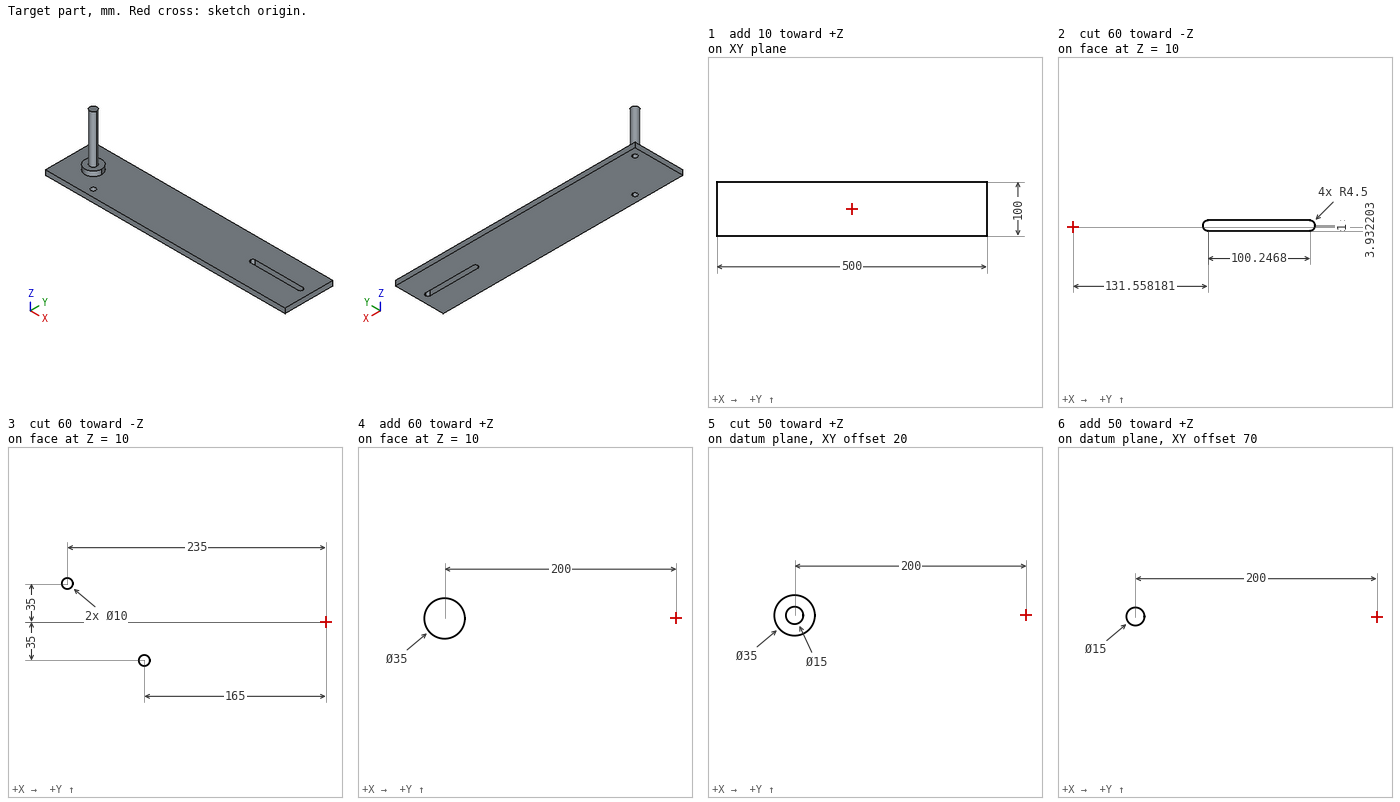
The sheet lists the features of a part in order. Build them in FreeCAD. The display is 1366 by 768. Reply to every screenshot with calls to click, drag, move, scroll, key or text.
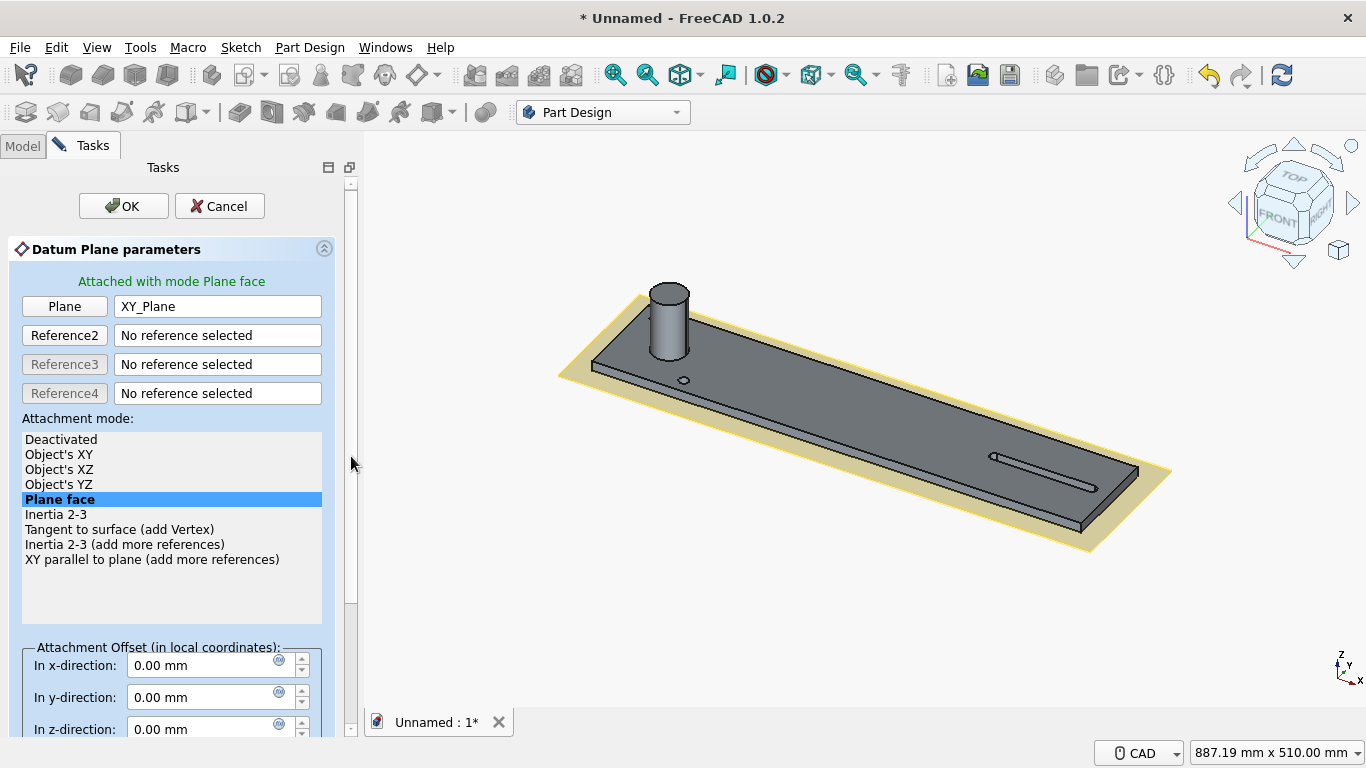
triple_click(210, 609)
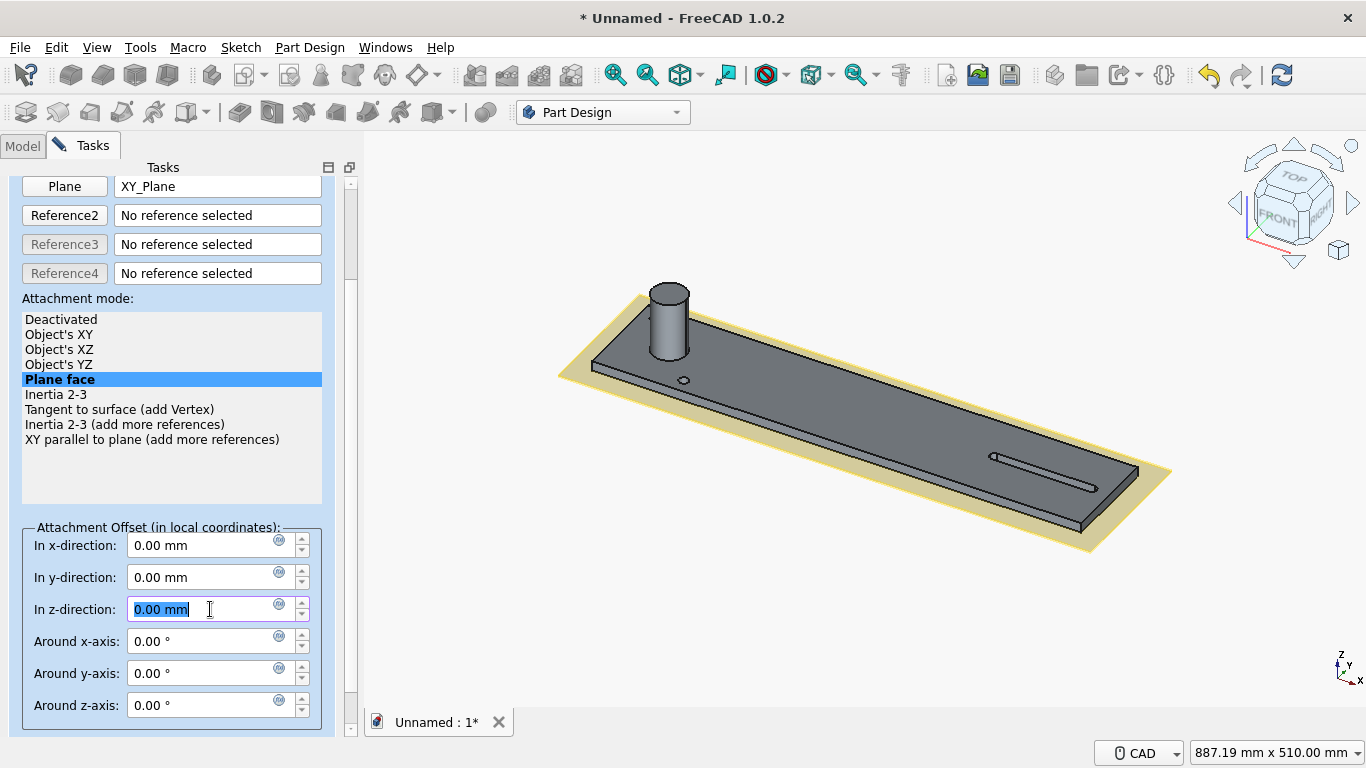
text(20)
key(Tab)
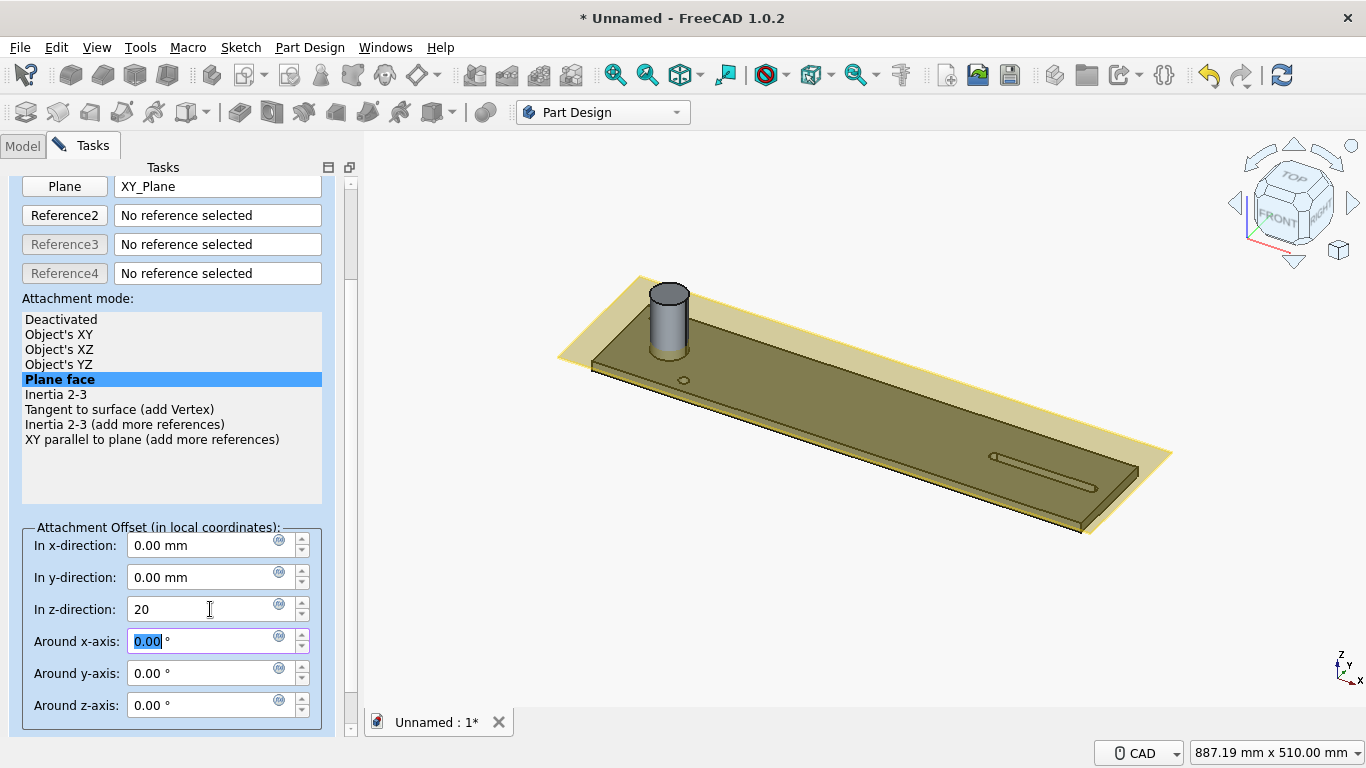
scroll(351, 456, up, 3)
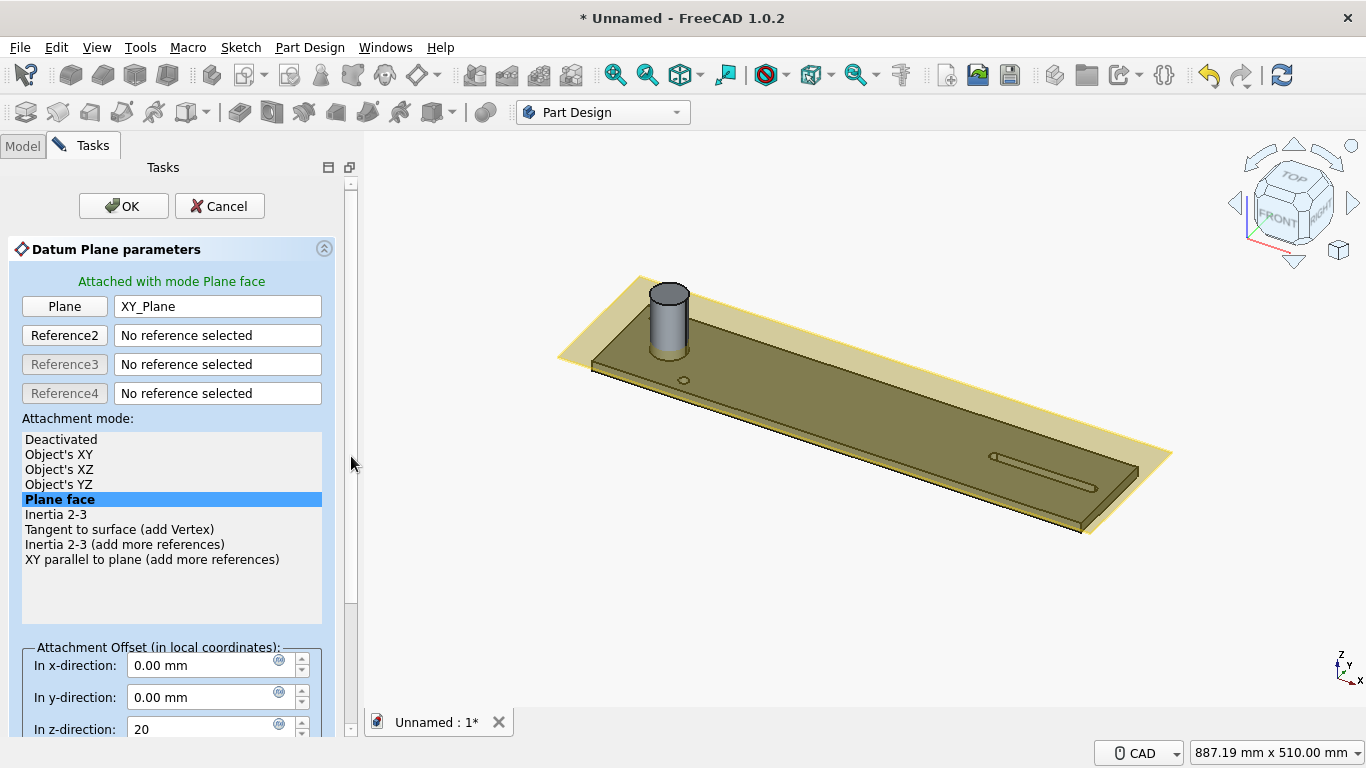
click(124, 206)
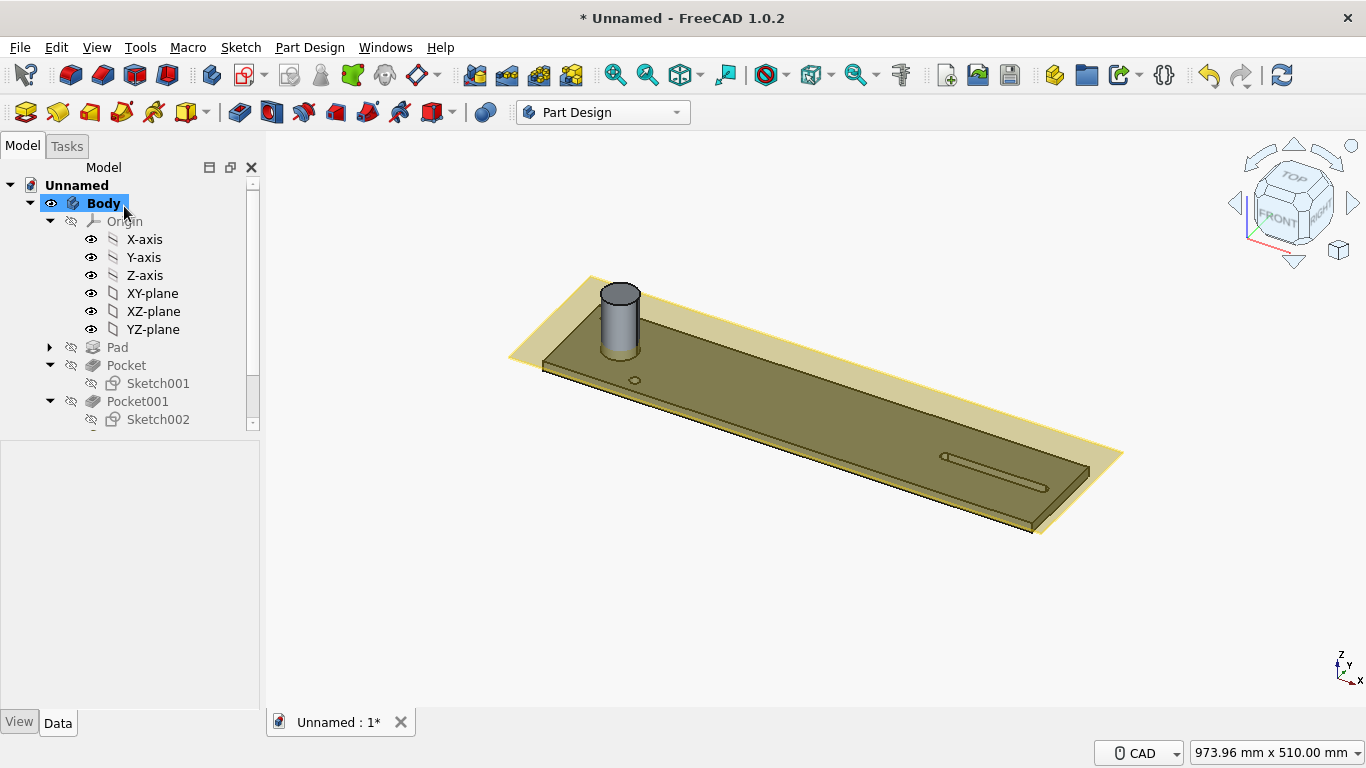
scroll(100, 307, down, 3)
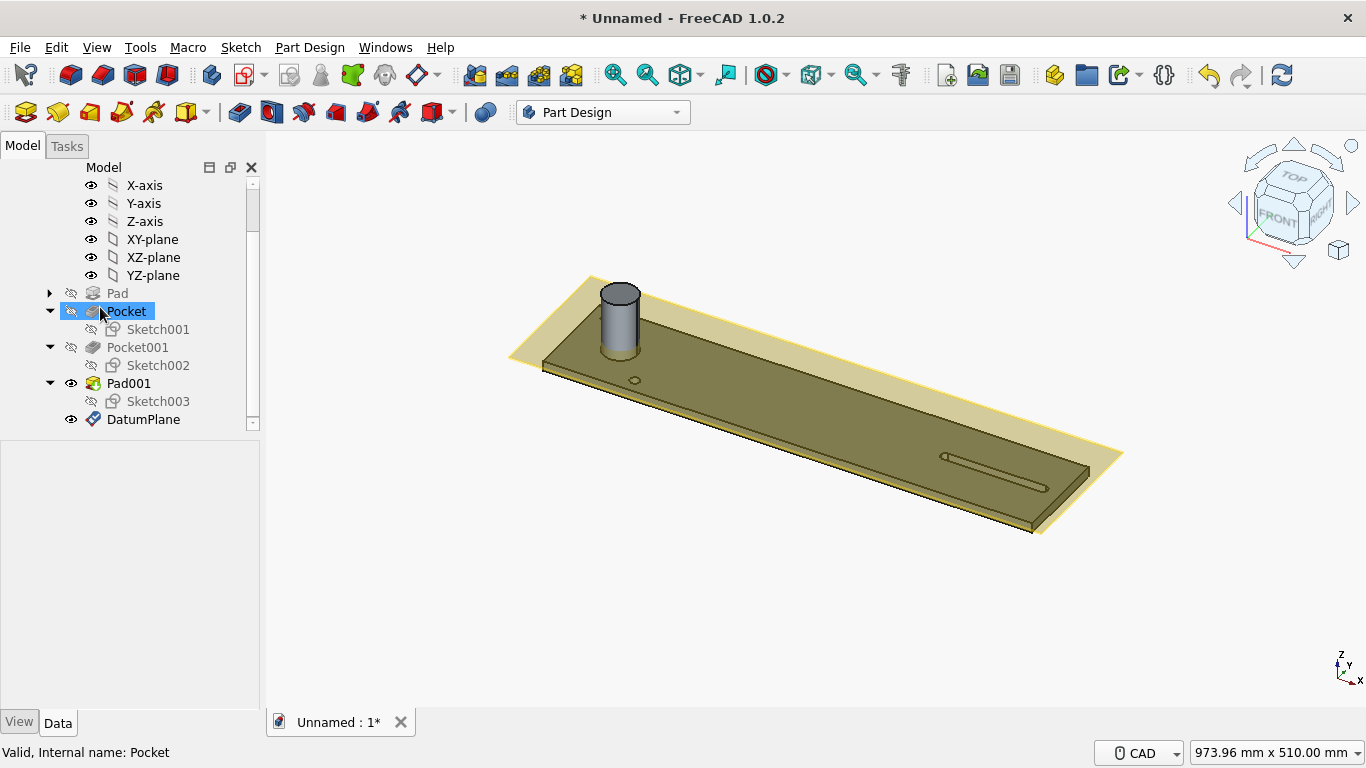
click(116, 419)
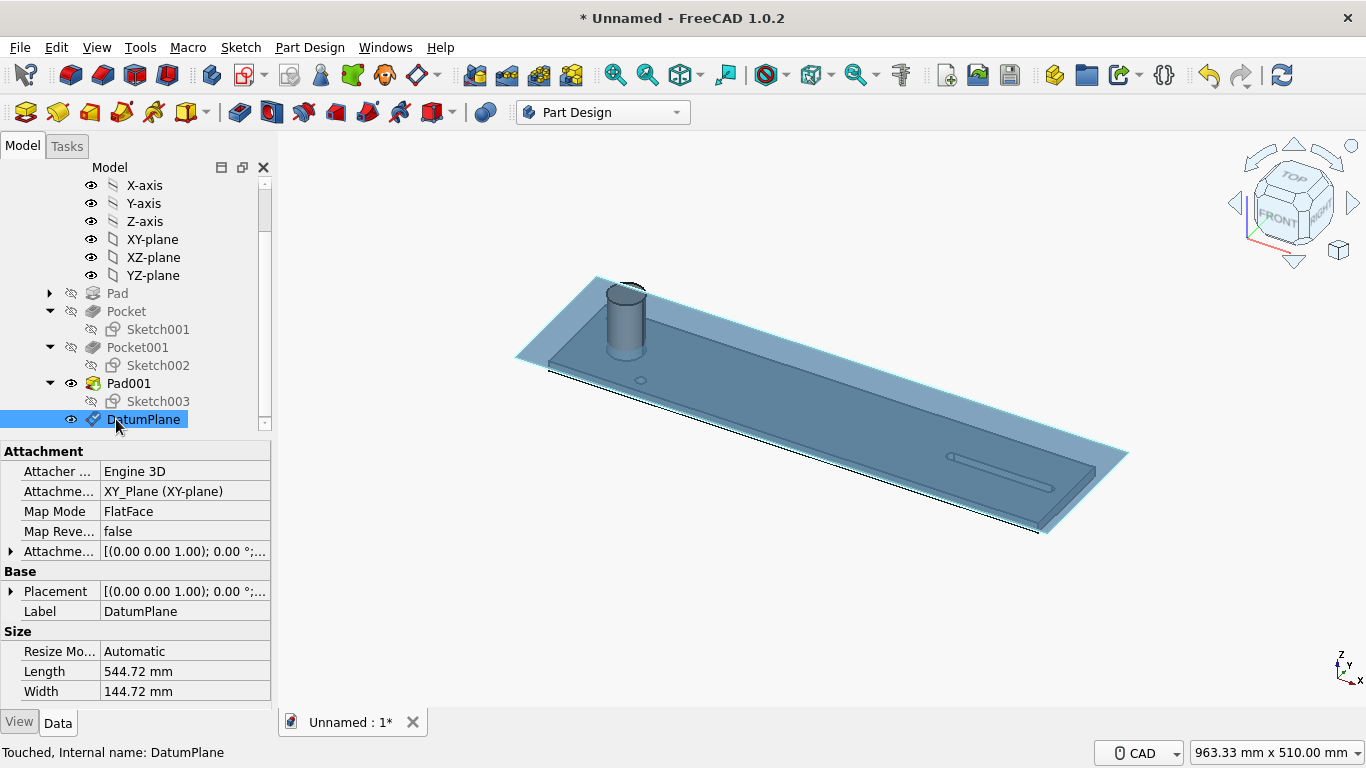
click(244, 76)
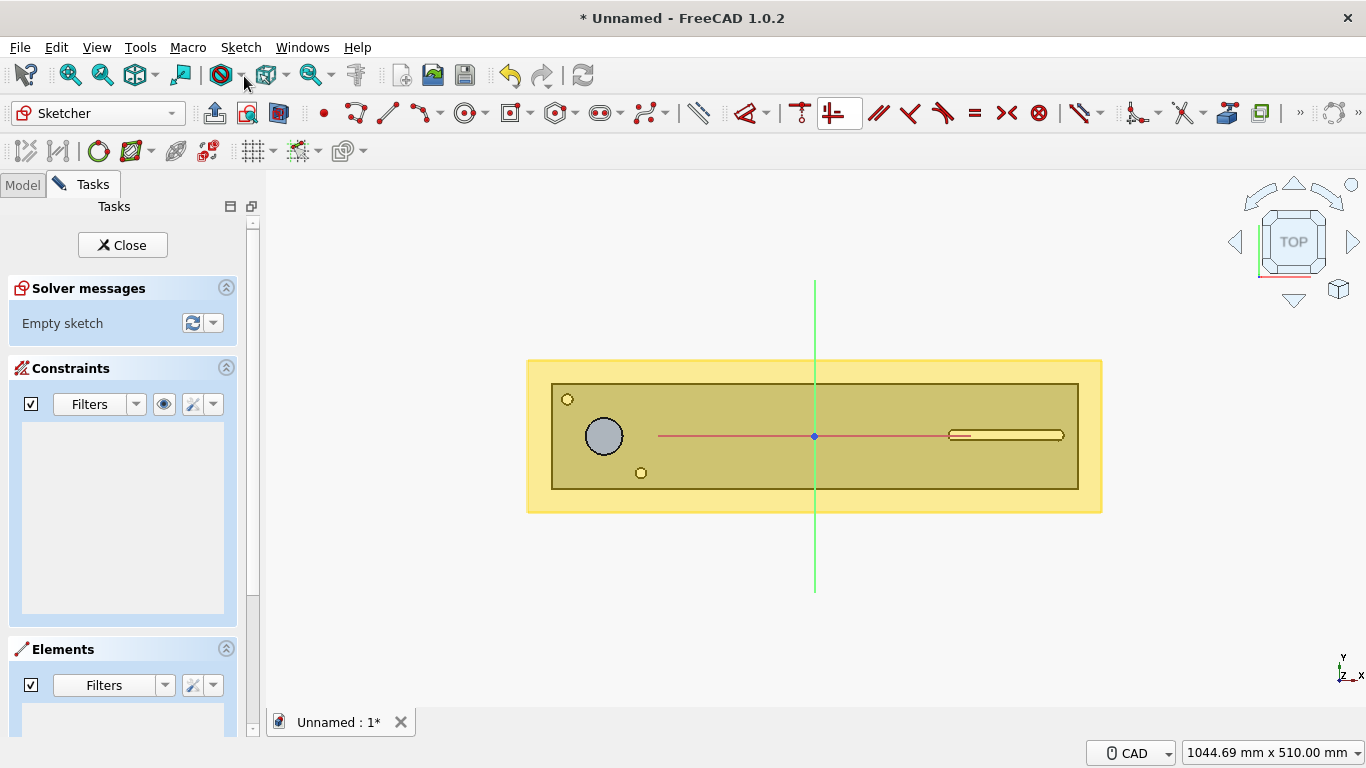
key(q)
key(s)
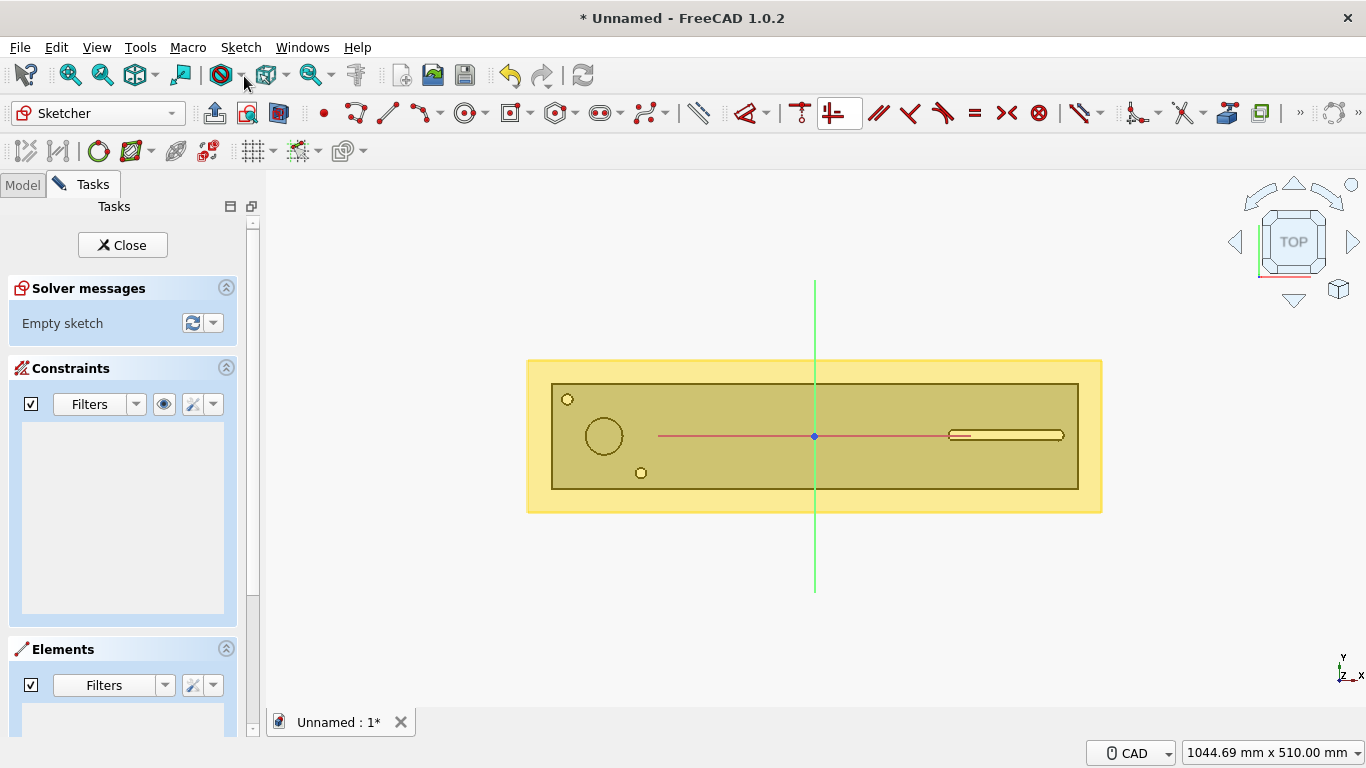
scroll(586, 436, up, 11)